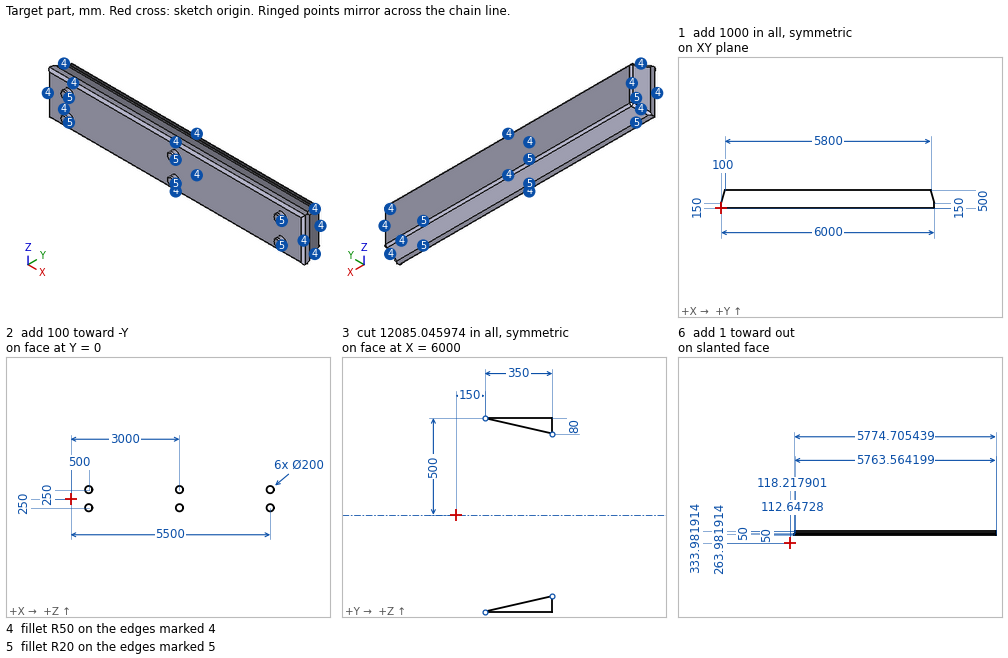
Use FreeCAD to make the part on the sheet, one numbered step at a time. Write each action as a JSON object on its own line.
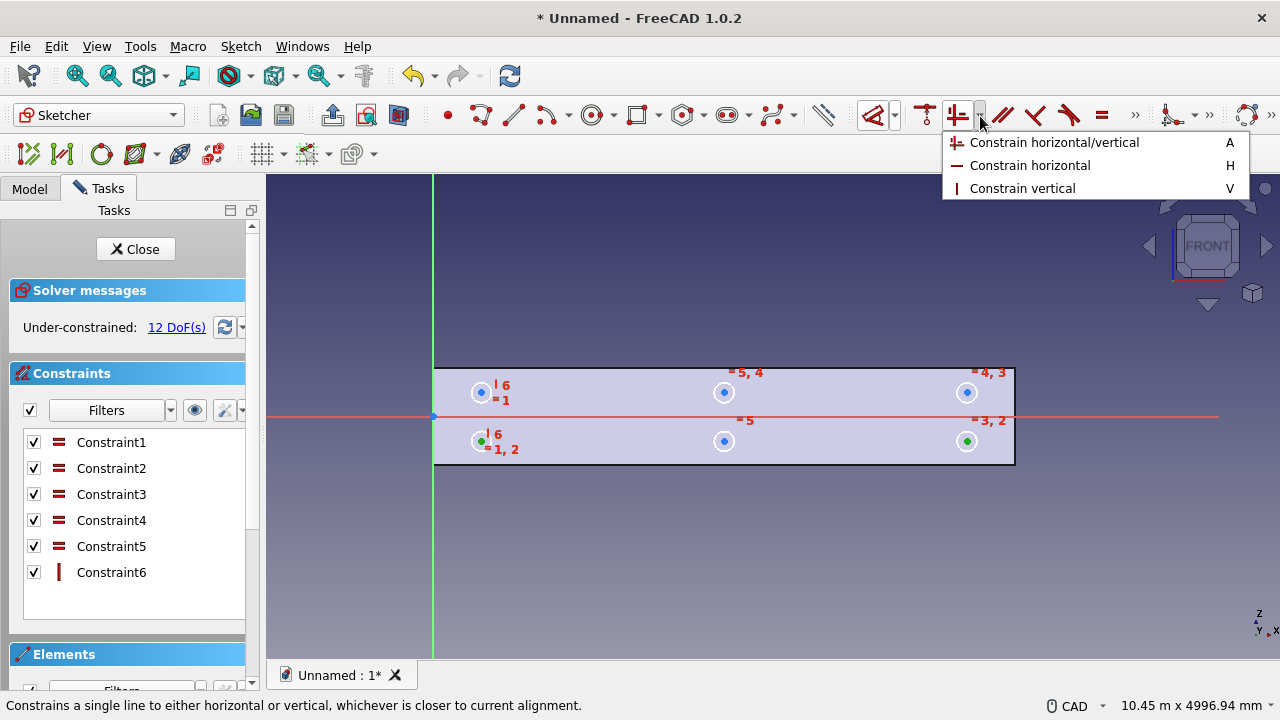
{"action": "left_click", "coordinate": [1096, 166]}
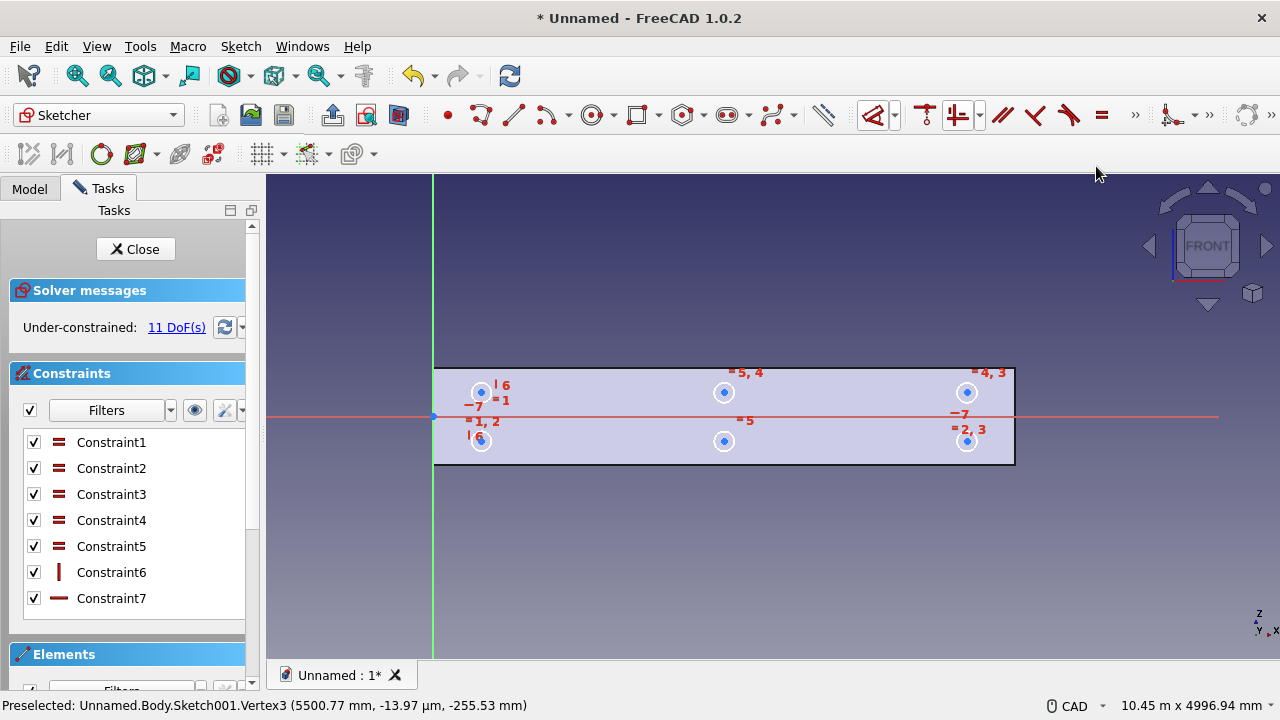
{"action": "left_click", "coordinate": [967, 441]}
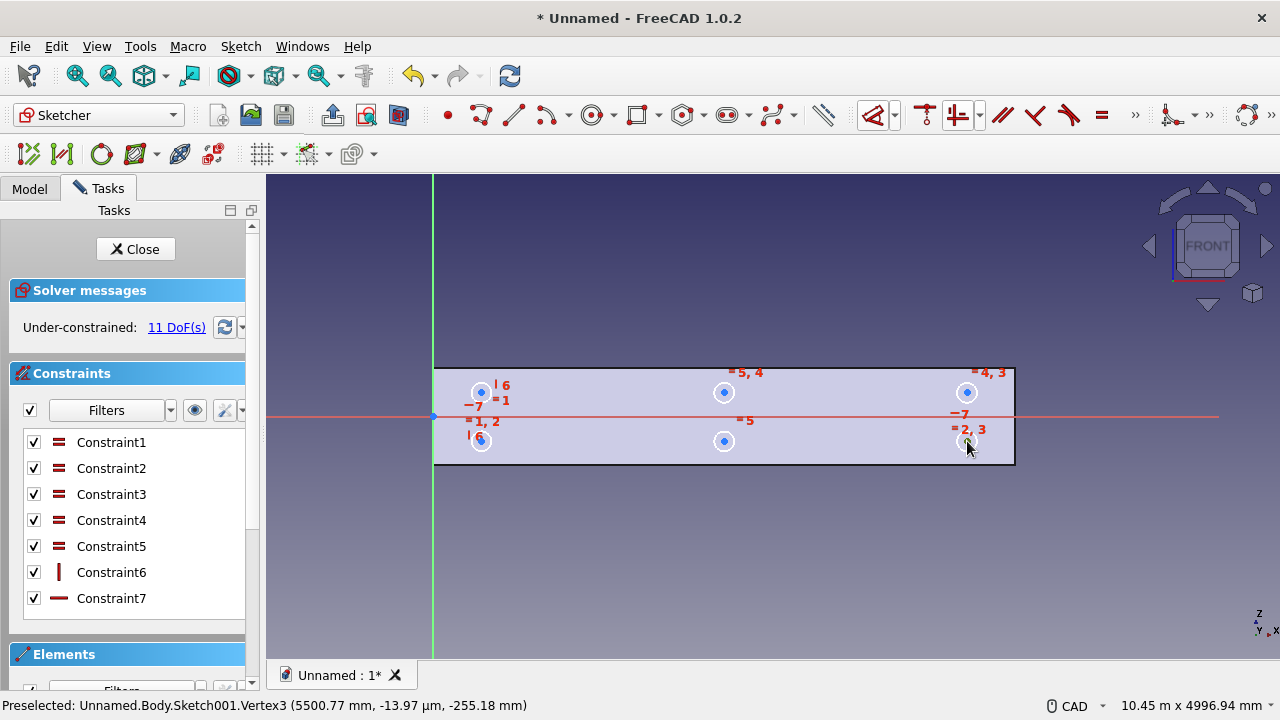
{"action": "left_click", "coordinate": [967, 393]}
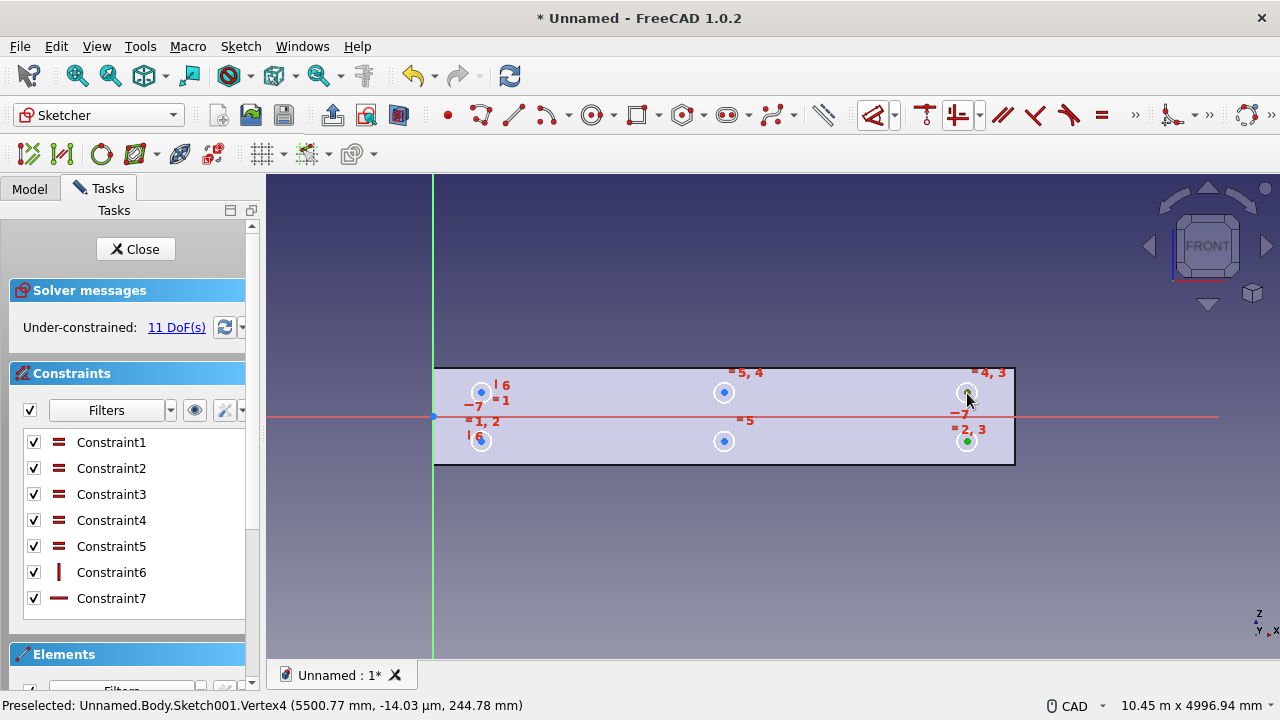
{"action": "key", "text": "v"}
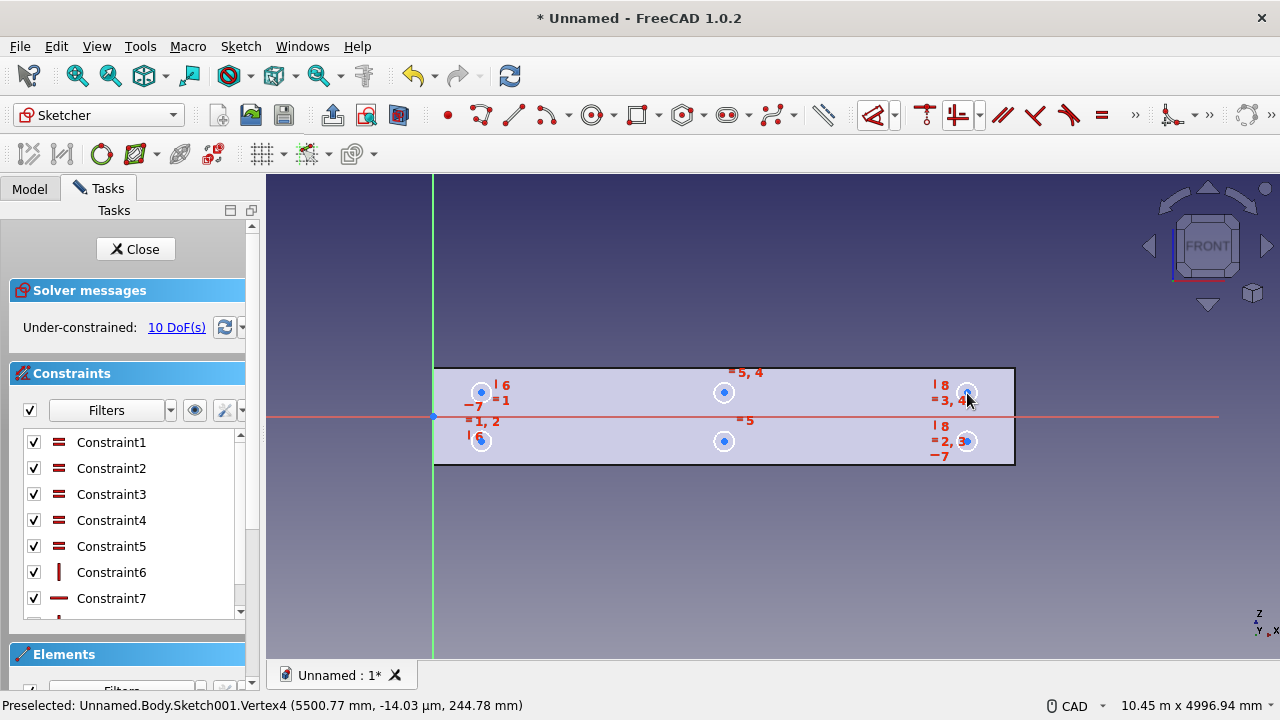
{"action": "left_click", "coordinate": [481, 393]}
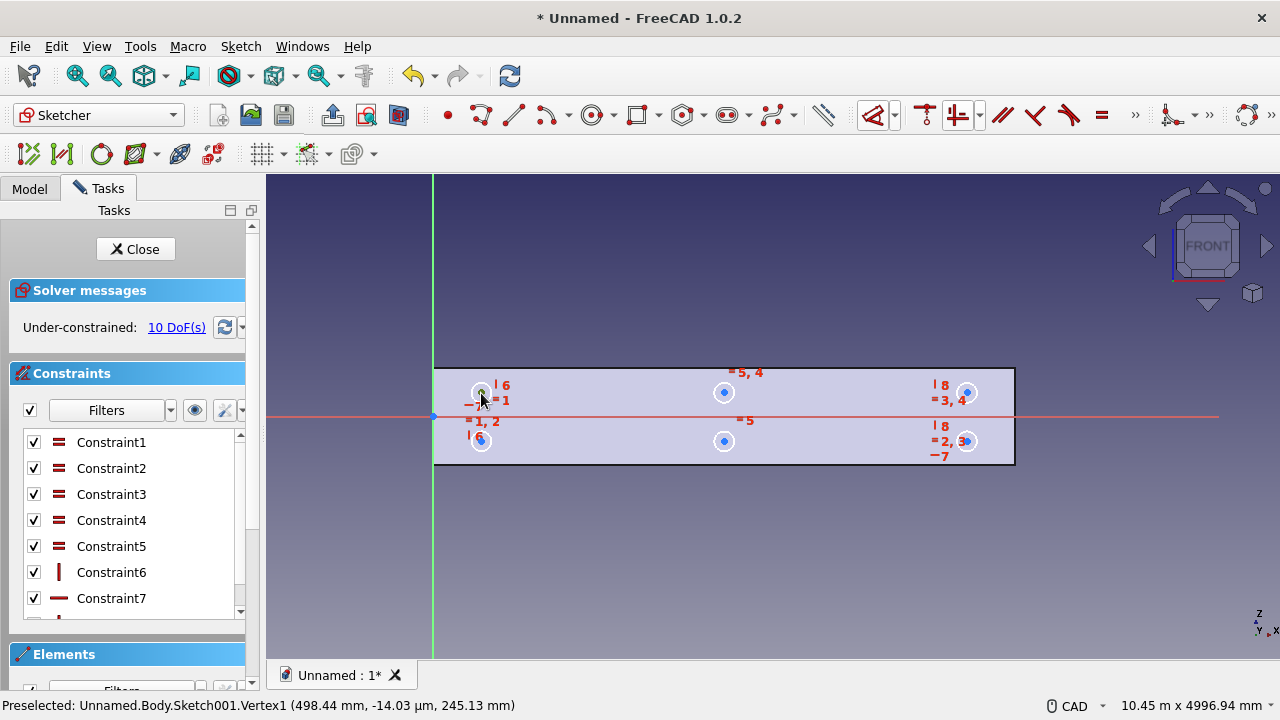
{"action": "left_click", "coordinate": [967, 393]}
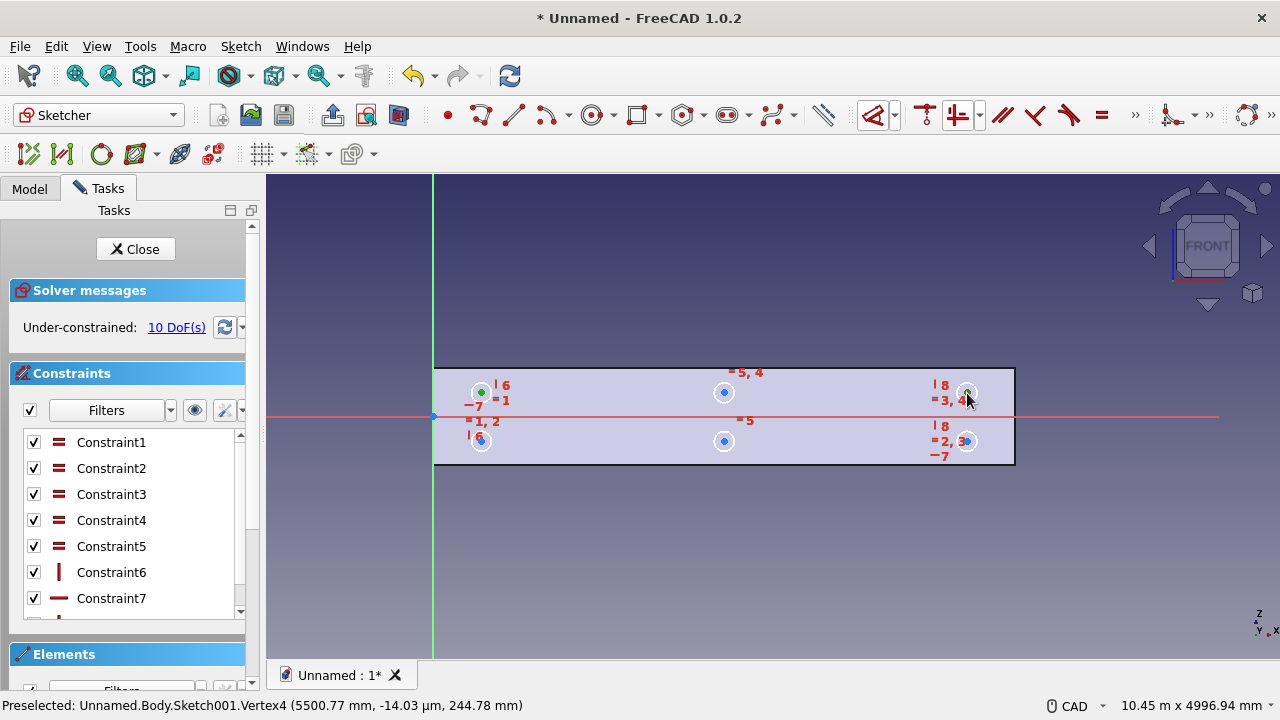
{"action": "left_click", "coordinate": [980, 116]}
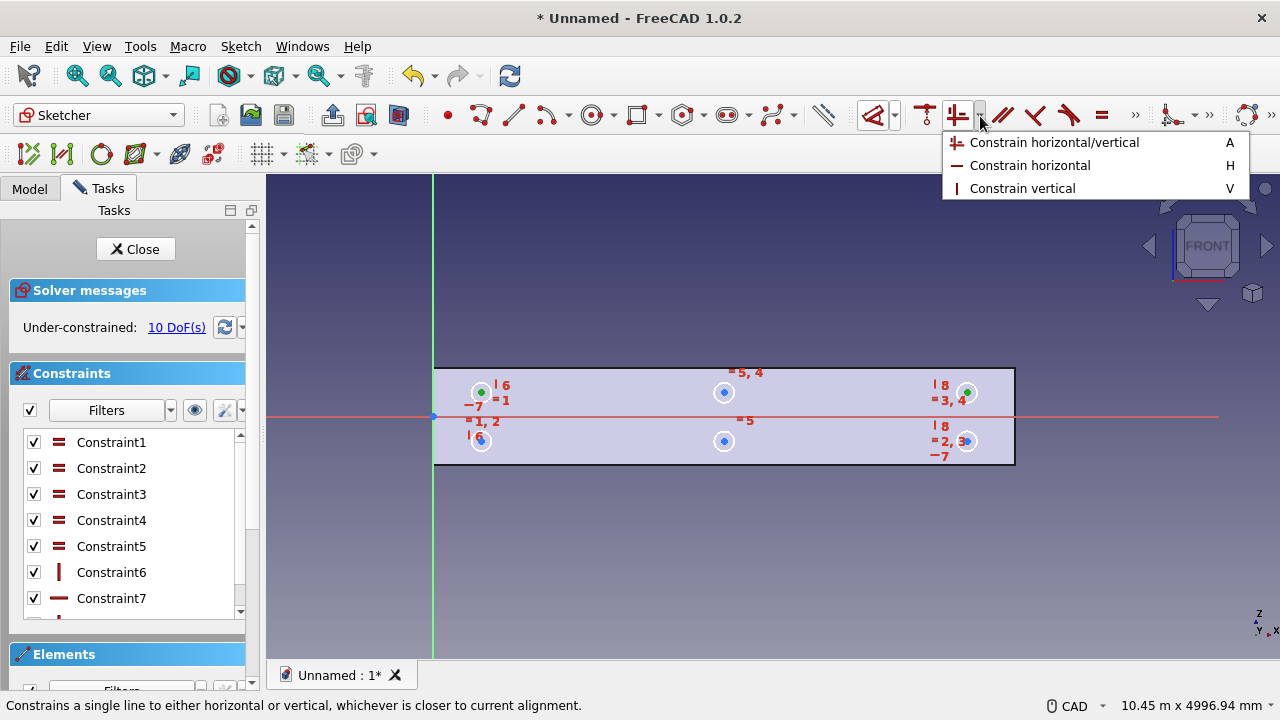
{"action": "left_click", "coordinate": [1096, 166]}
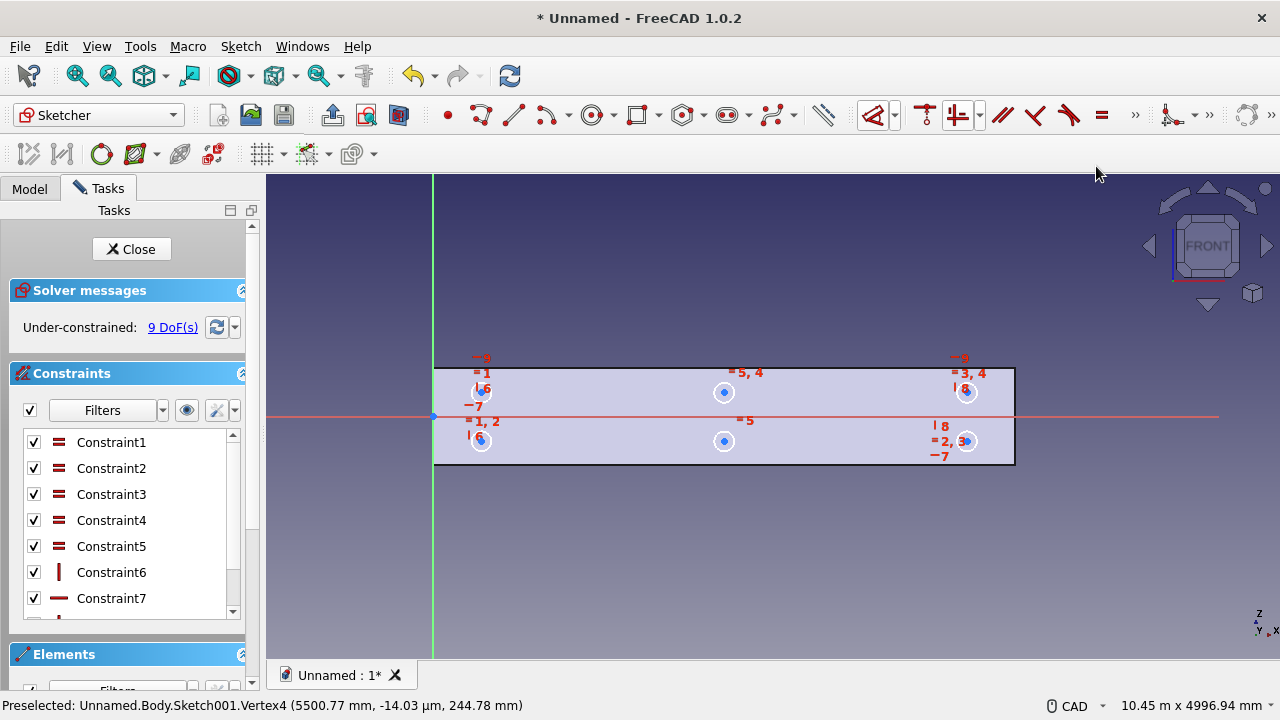
{"action": "left_click", "coordinate": [481, 393]}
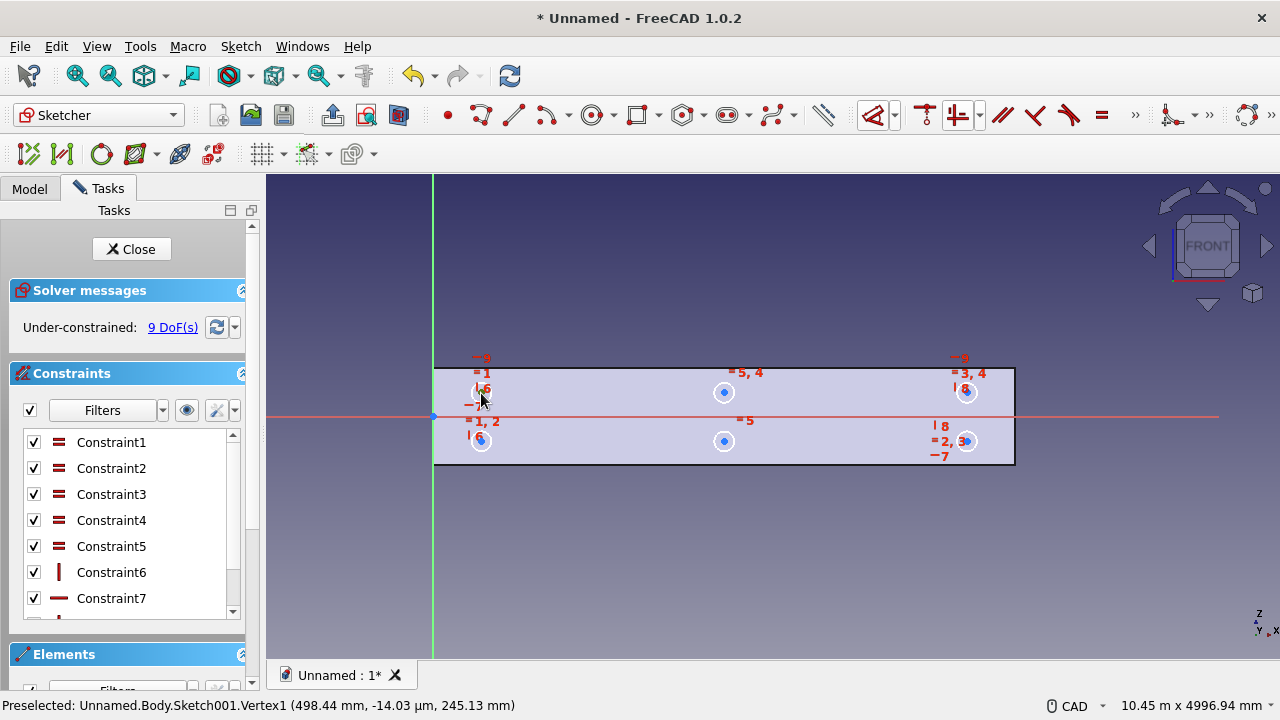
{"action": "left_click", "coordinate": [724, 393]}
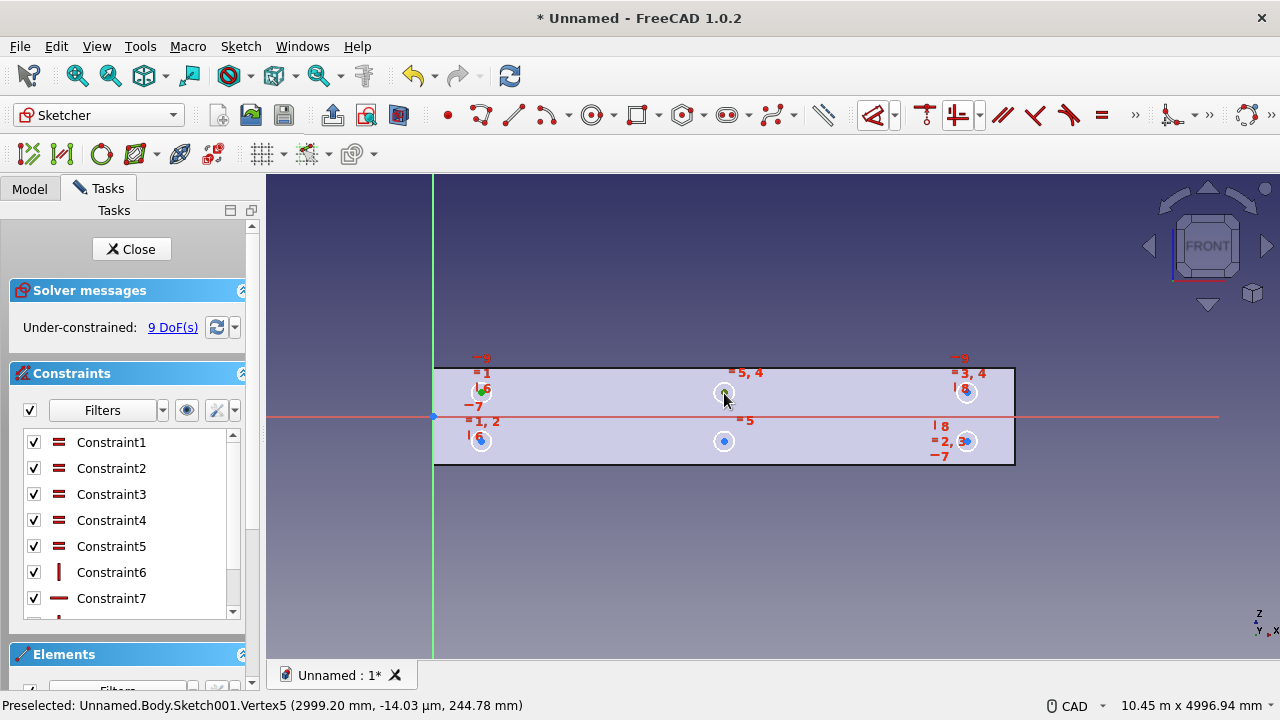
{"action": "left_click", "coordinate": [980, 116]}